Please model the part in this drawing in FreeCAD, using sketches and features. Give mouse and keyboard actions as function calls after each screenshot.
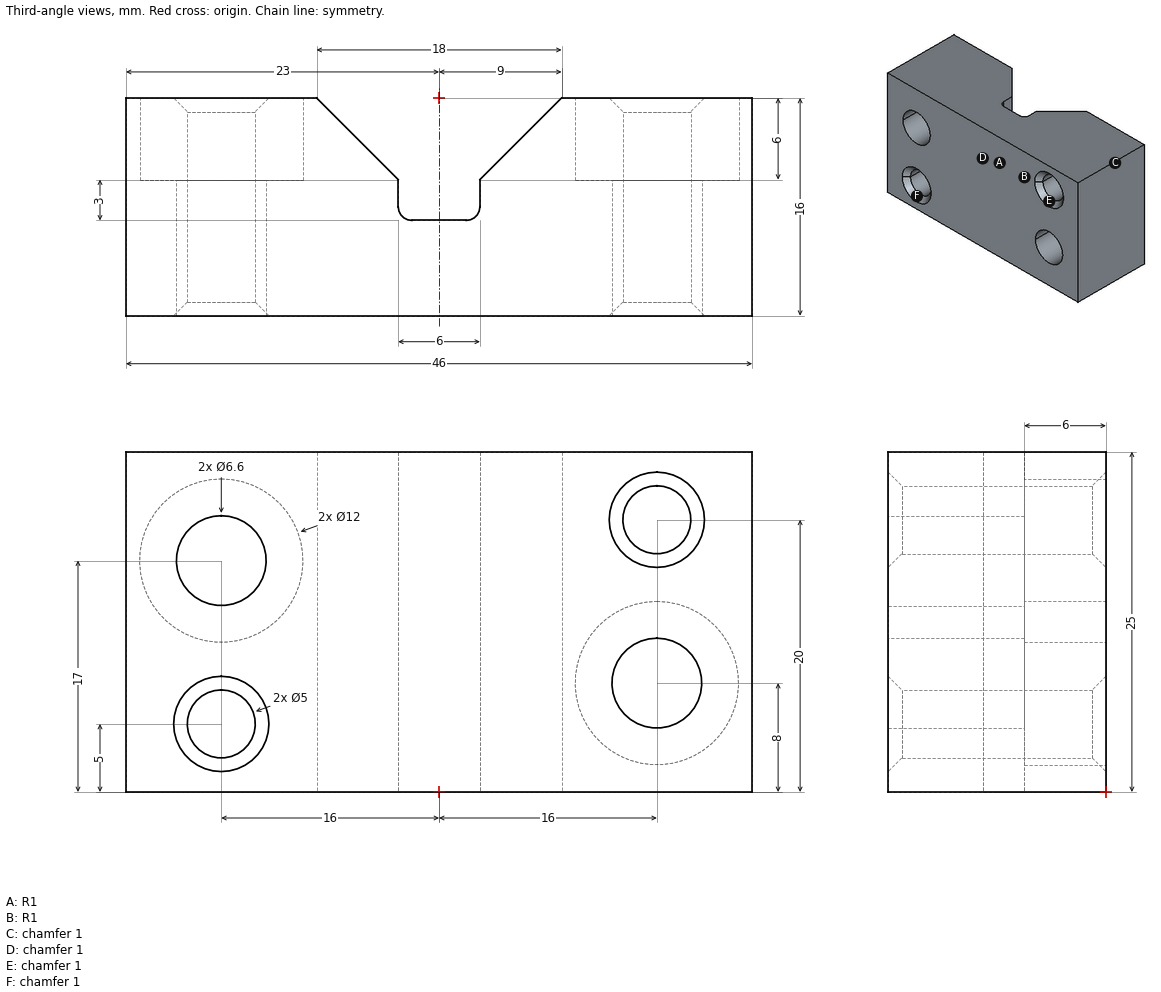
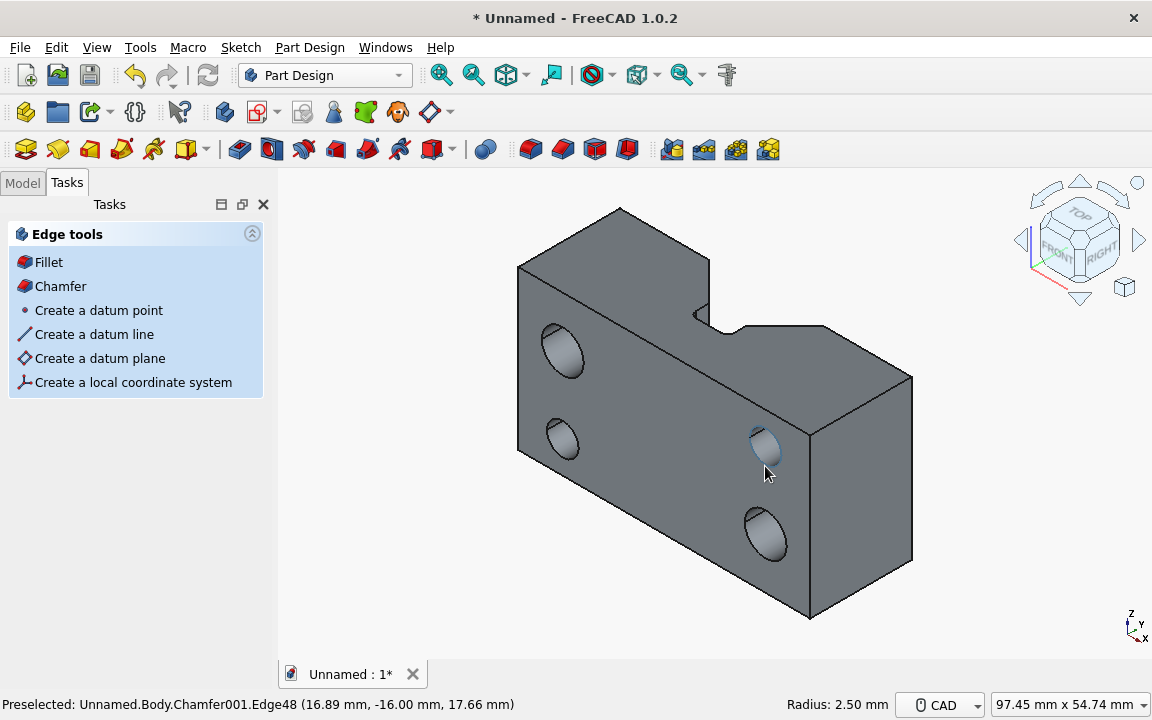
click(564, 150)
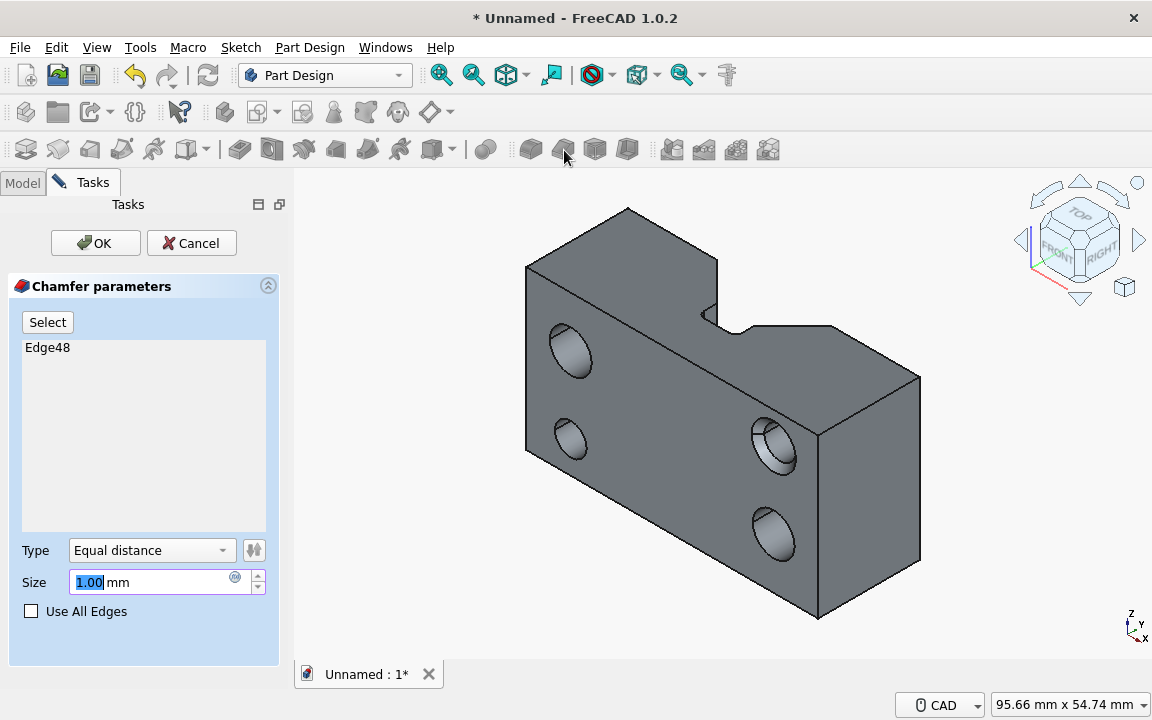
text(1)
key(Tab)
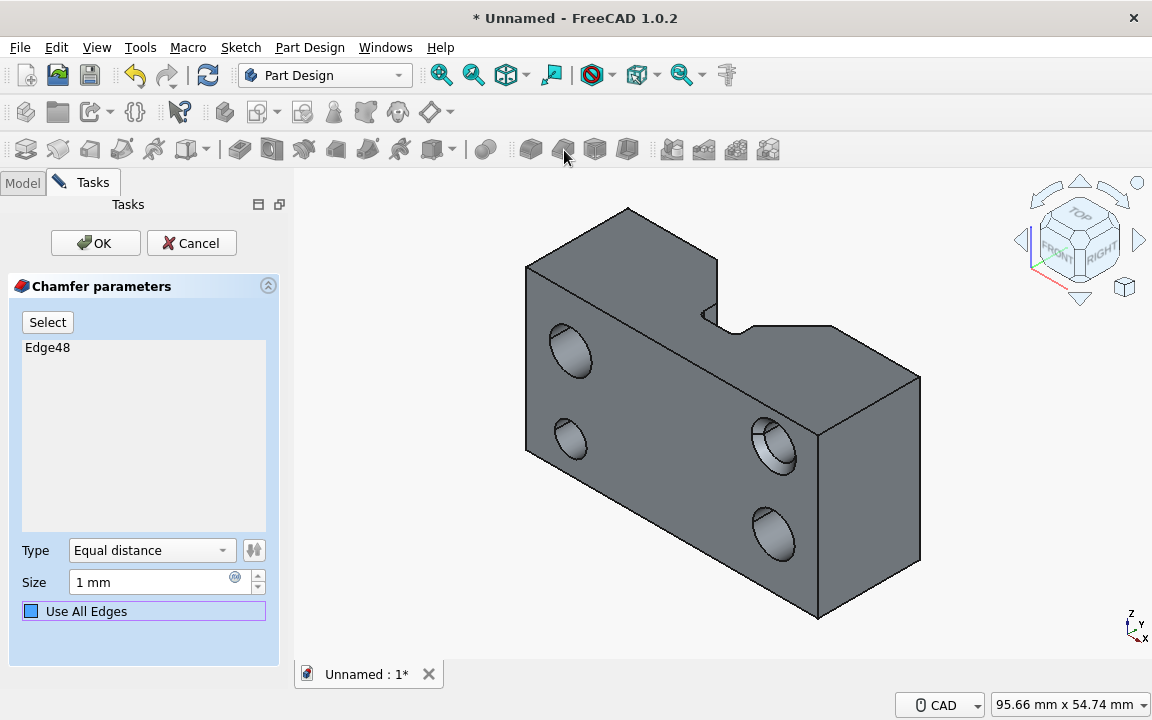
click(96, 243)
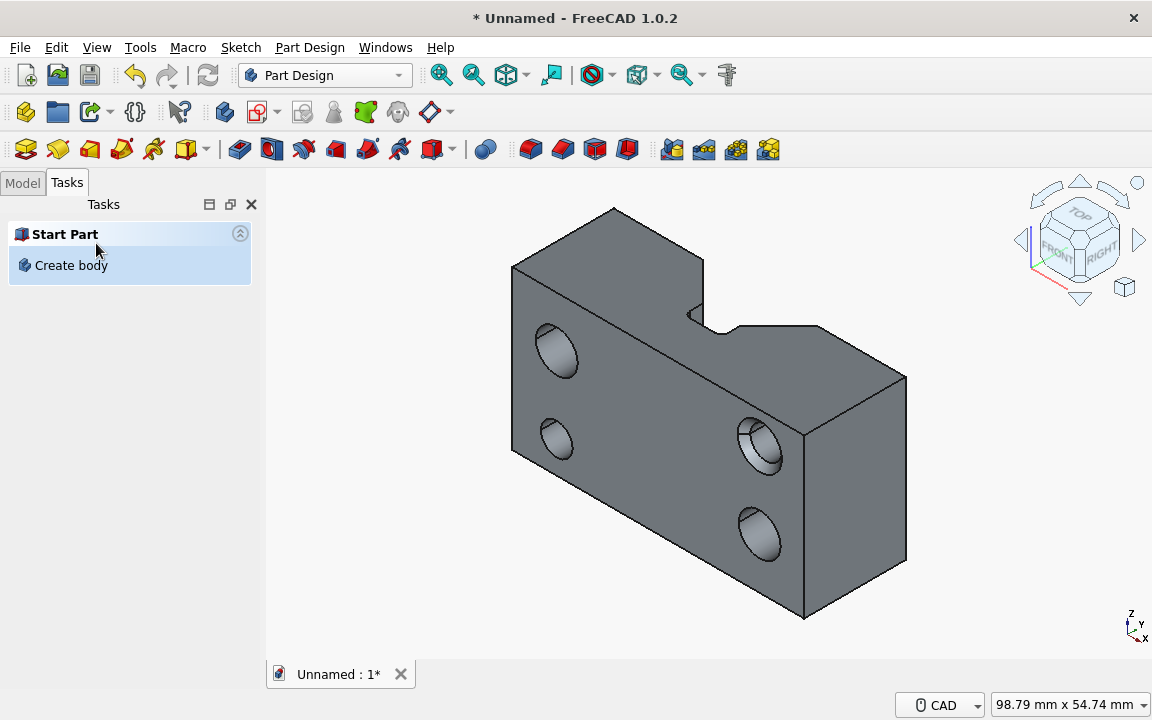
click(570, 456)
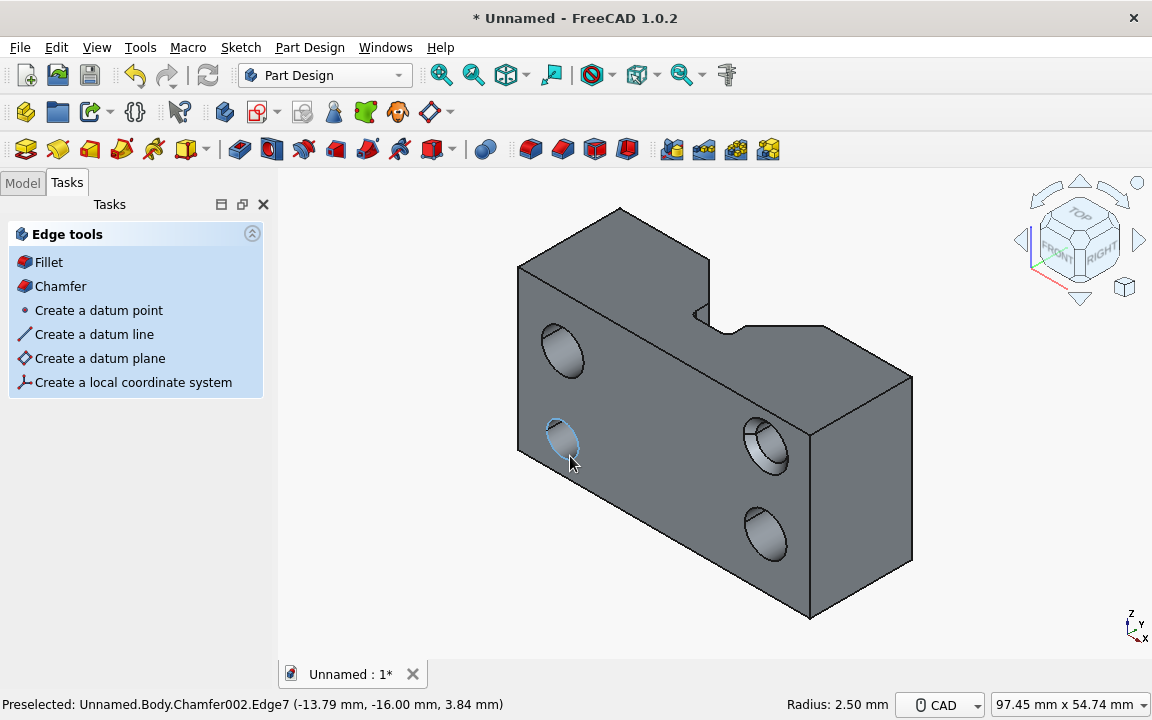
click(564, 150)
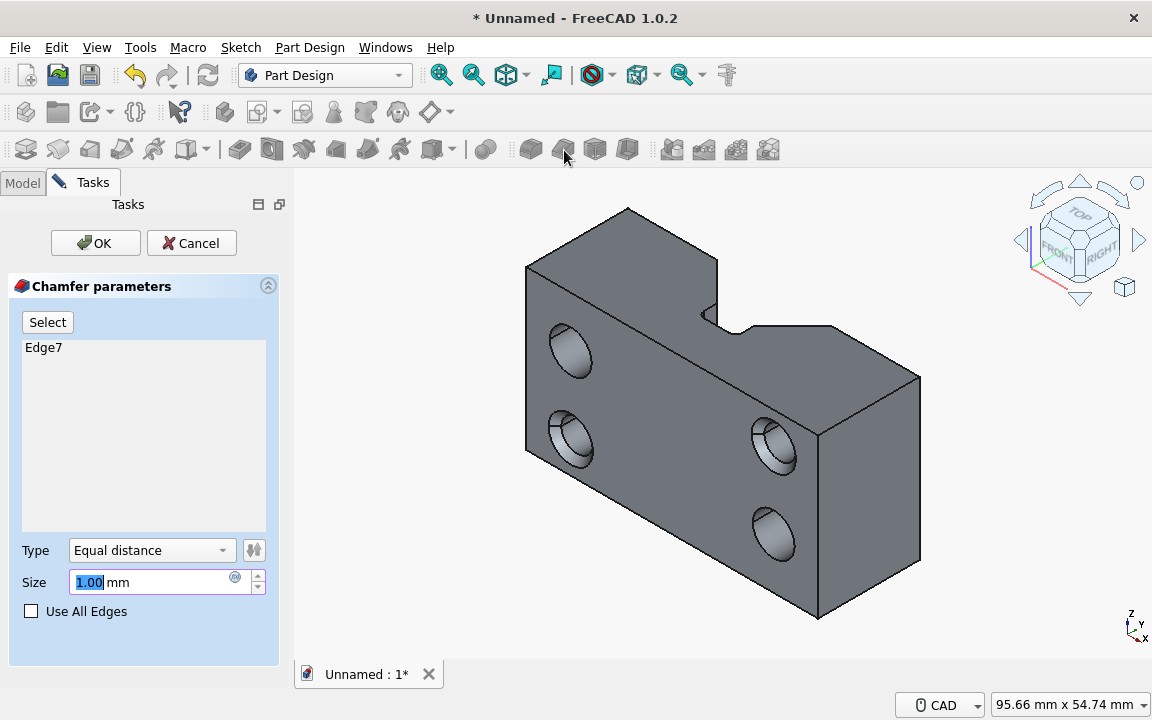
text(1)
key(Tab)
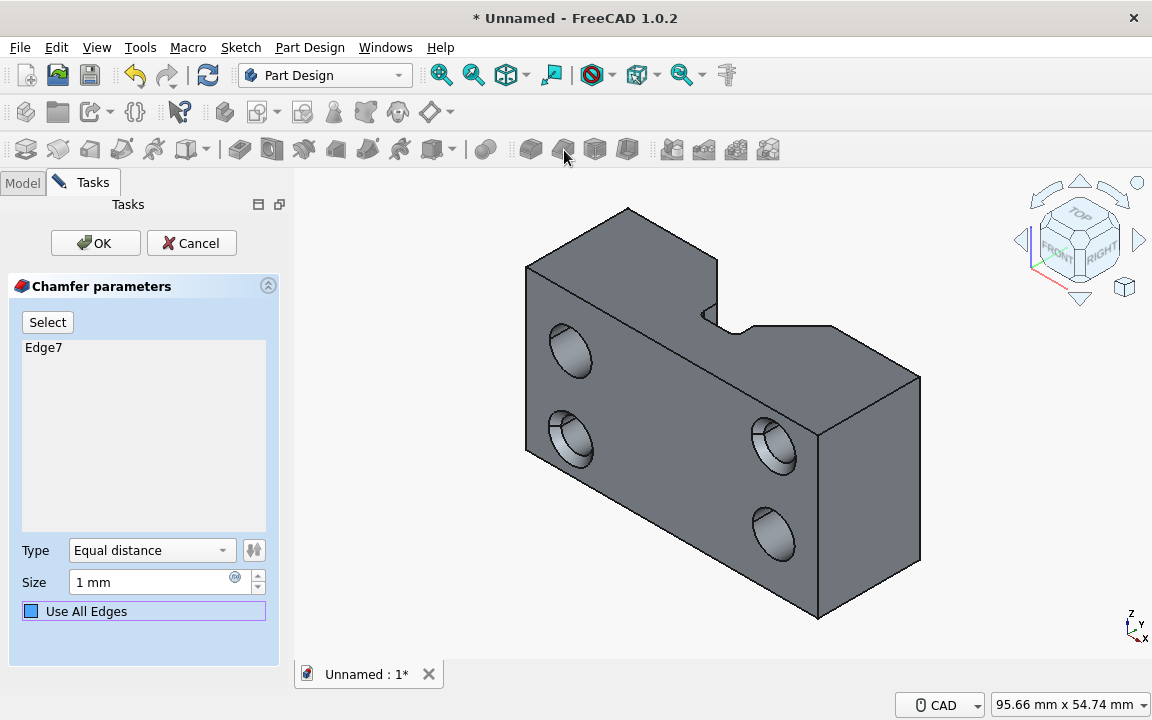
click(96, 243)